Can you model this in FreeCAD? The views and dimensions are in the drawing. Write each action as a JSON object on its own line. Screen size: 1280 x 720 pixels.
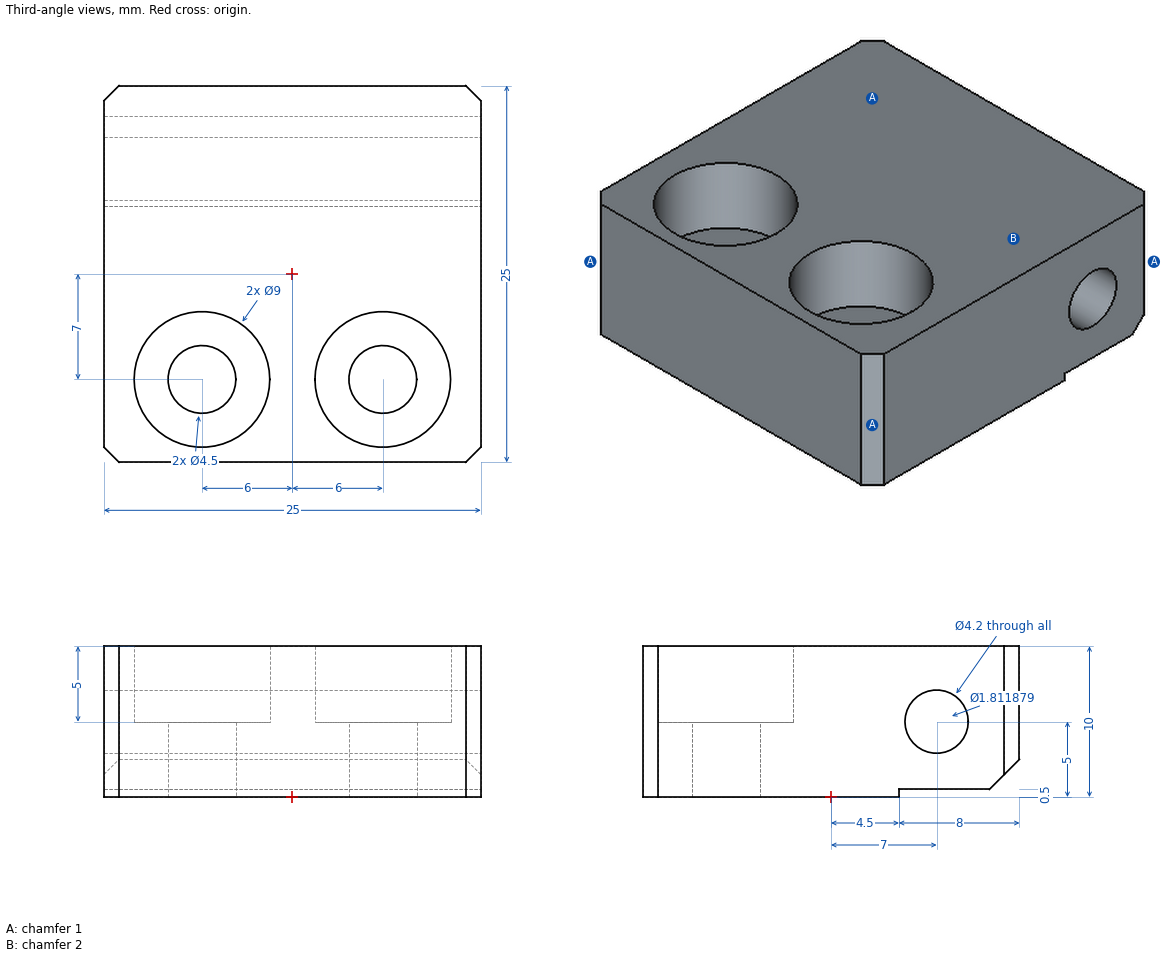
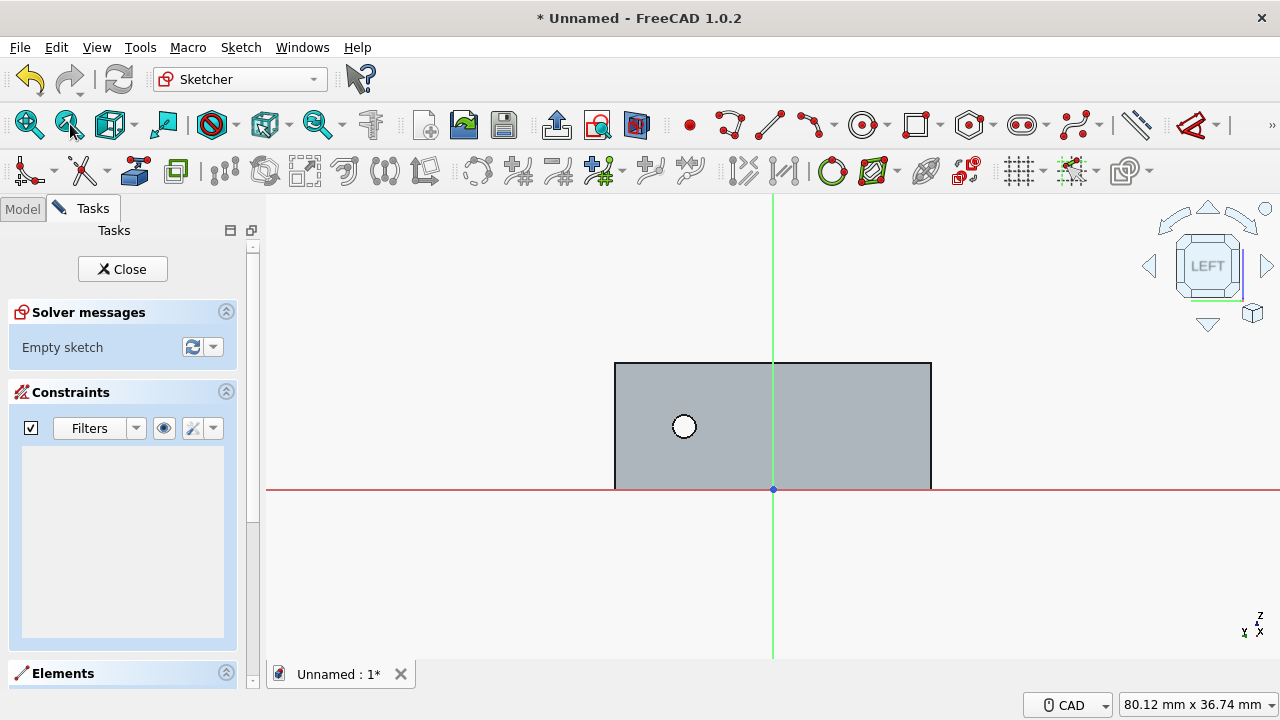
{"action": "scroll", "coordinate": [720, 453], "scroll_direction": "up", "scroll_amount": 6}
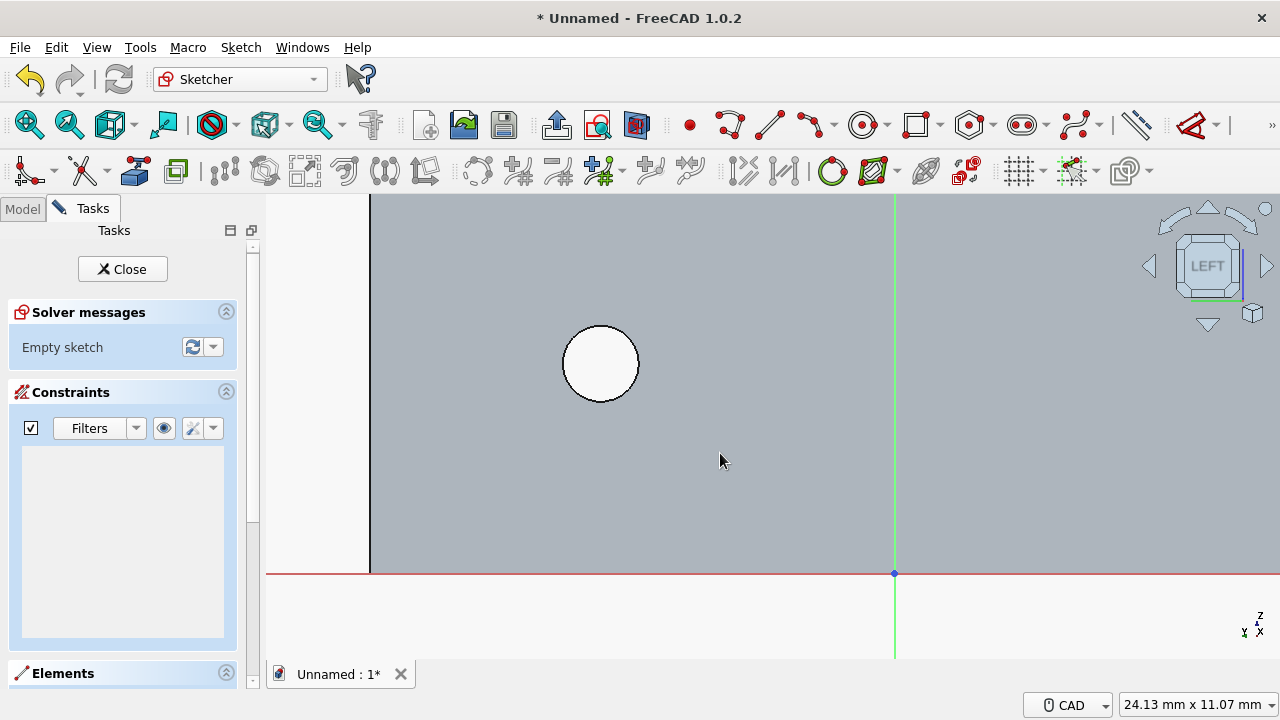
{"action": "key", "text": "g c"}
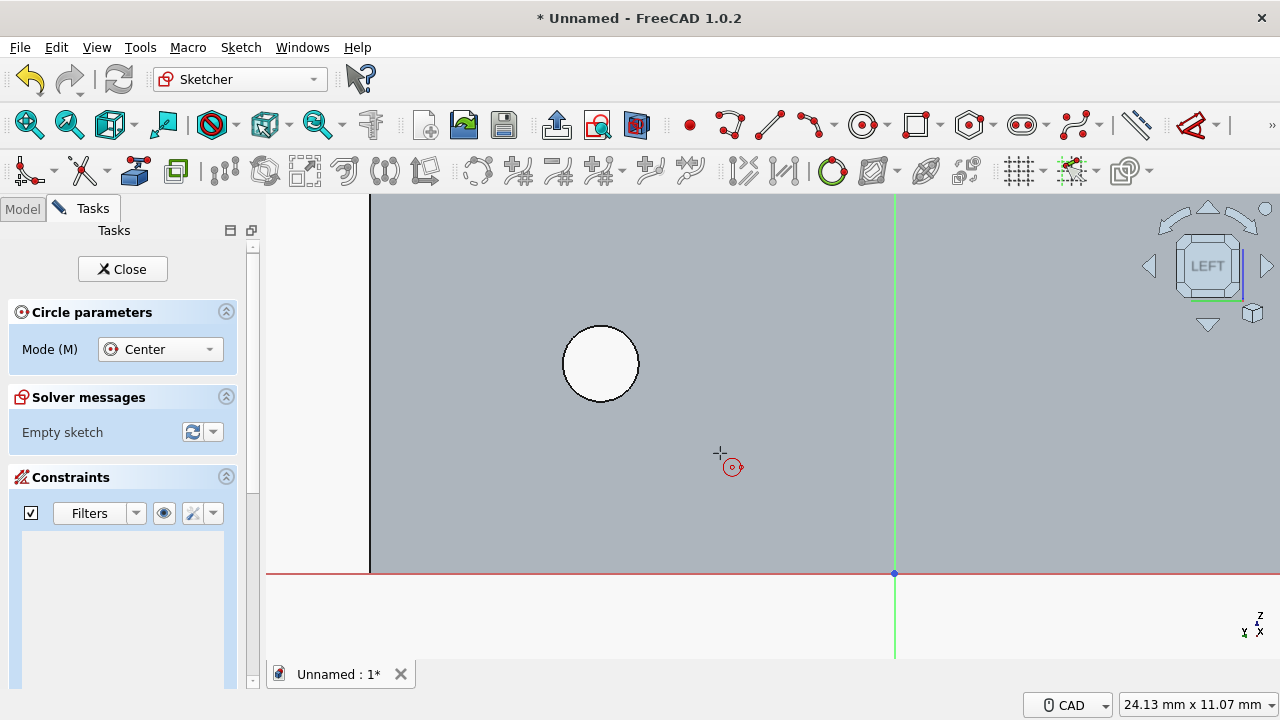
{"action": "left_click", "coordinate": [601, 364]}
{"action": "left_click", "coordinate": [663, 301]}
{"action": "key", "text": "Escape"}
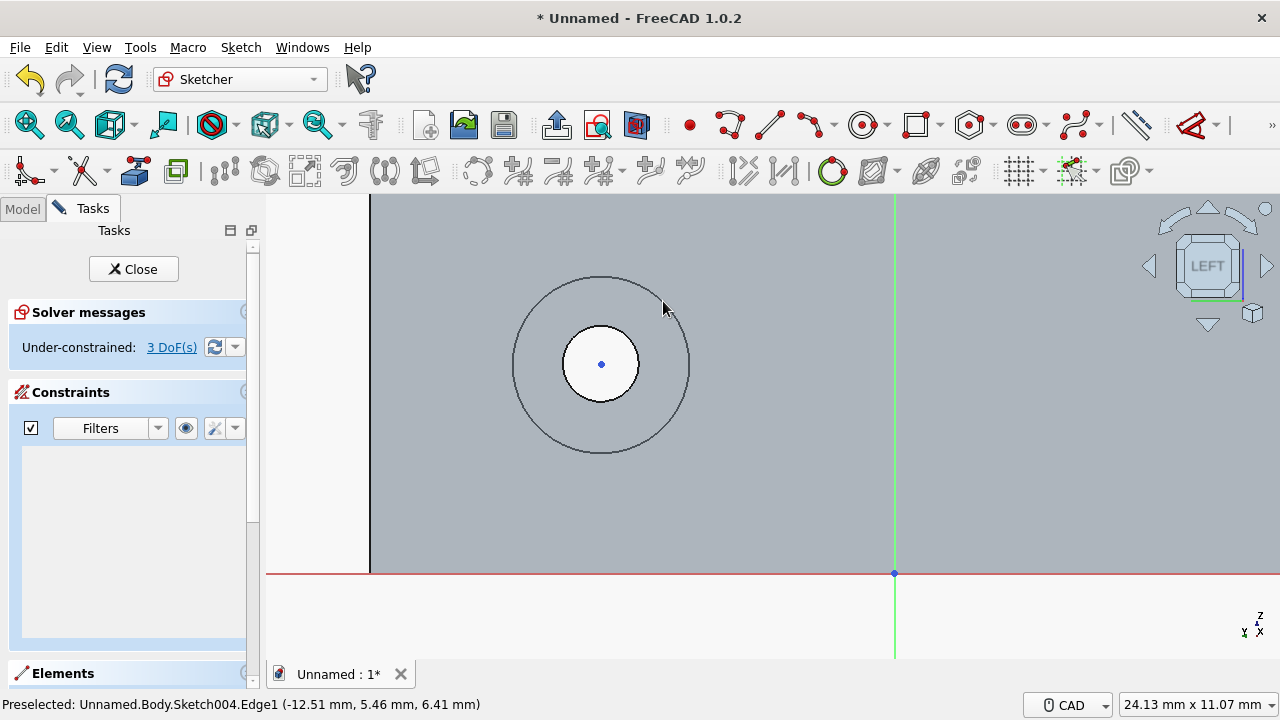
{"action": "key", "text": "d"}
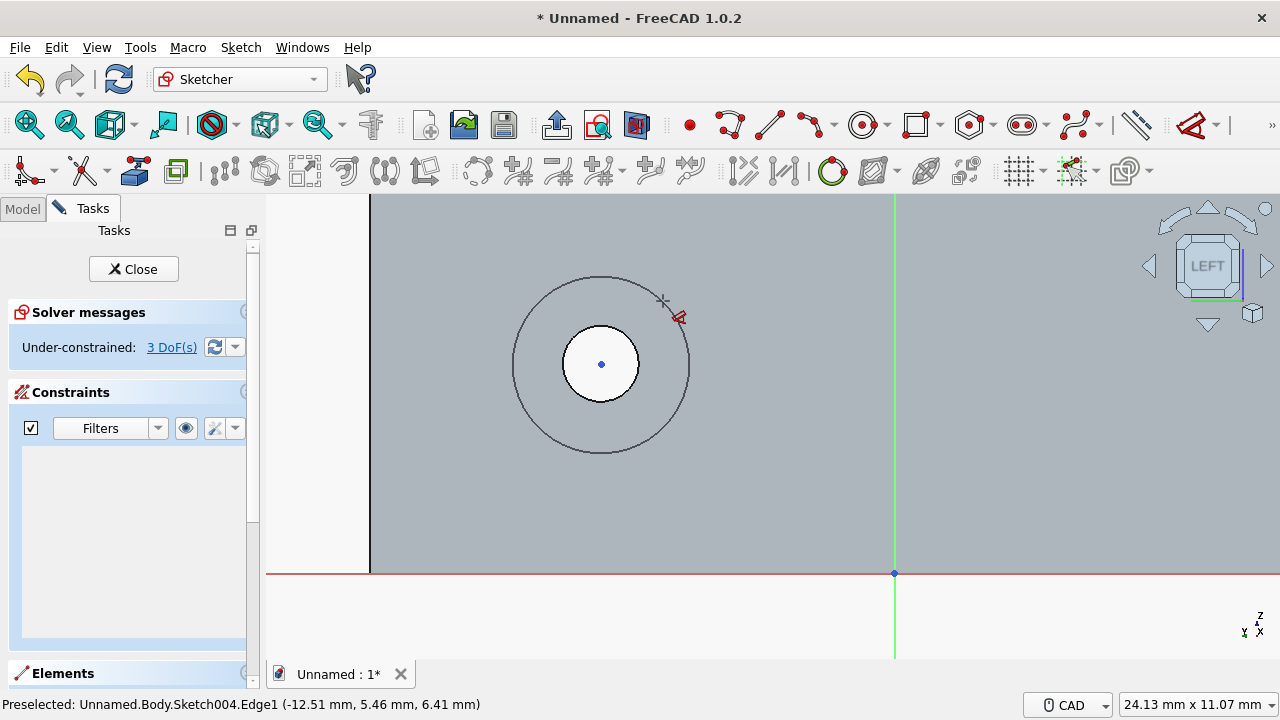
{"action": "left_click", "coordinate": [663, 302]}
{"action": "left_click", "coordinate": [685, 279]}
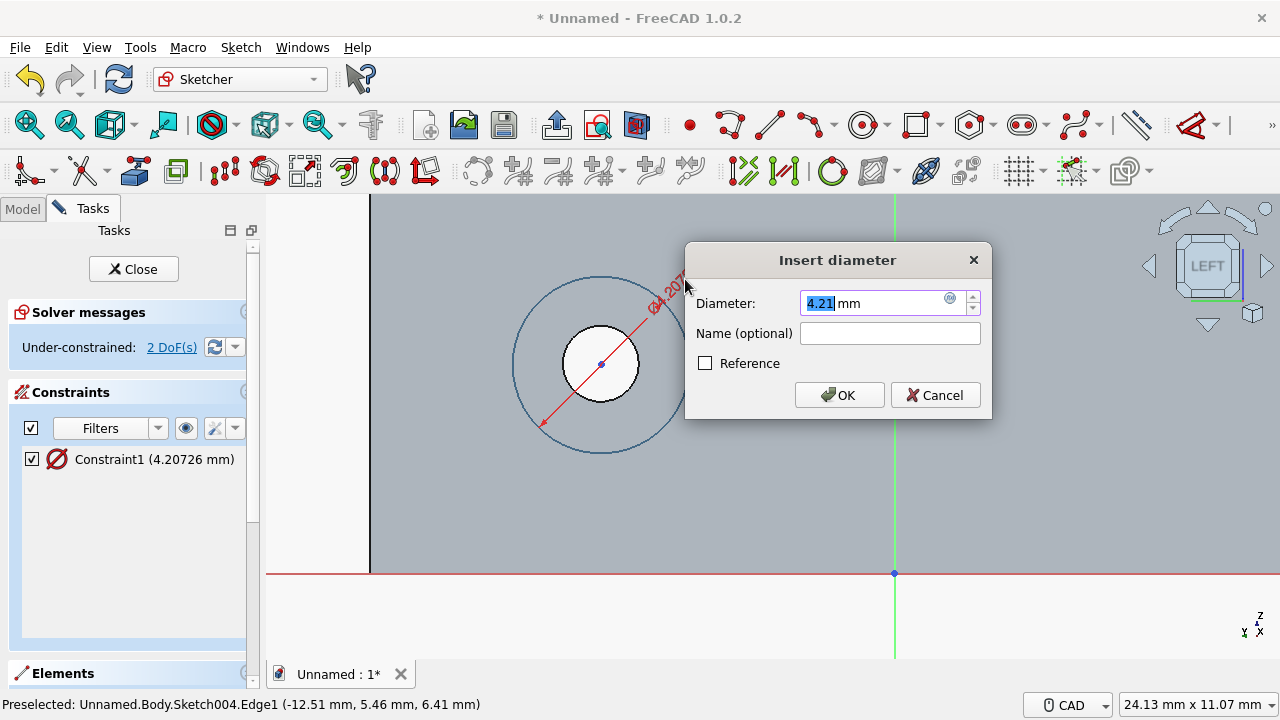
{"action": "type", "text": "4.2"}
{"action": "key", "text": "Return"}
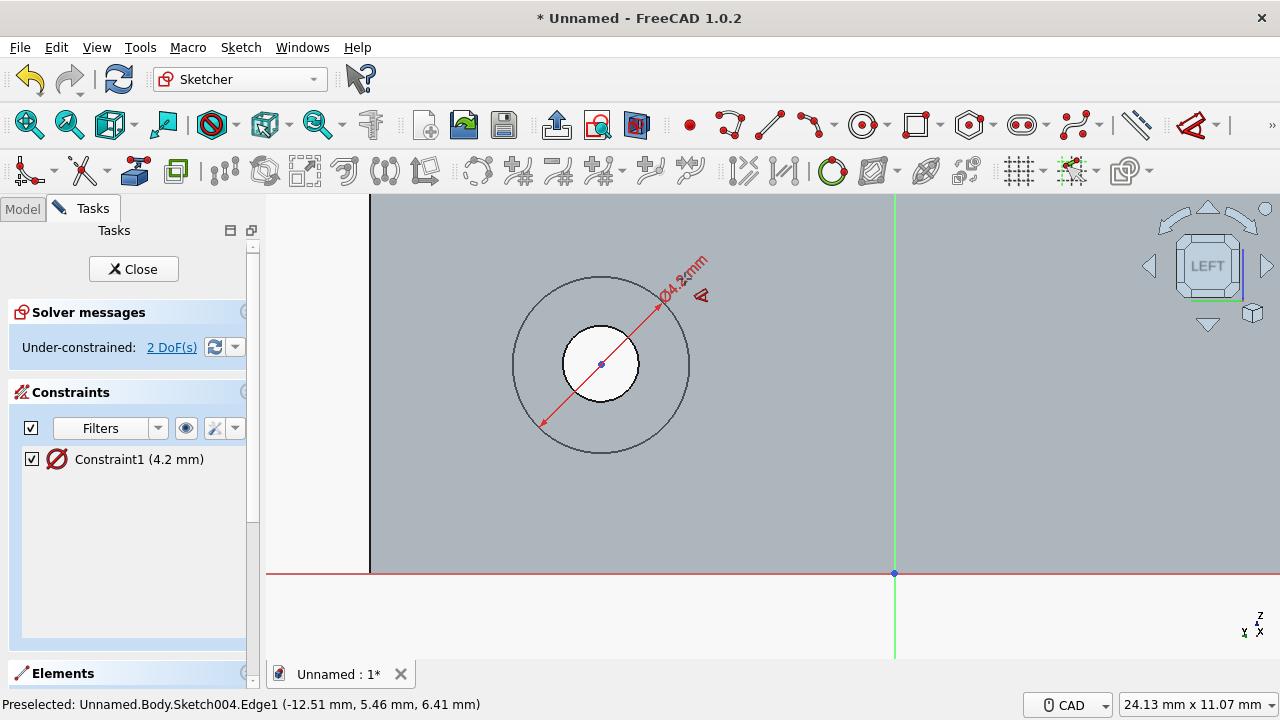
{"action": "left_click", "coordinate": [601, 365]}
{"action": "left_click", "coordinate": [748, 608]}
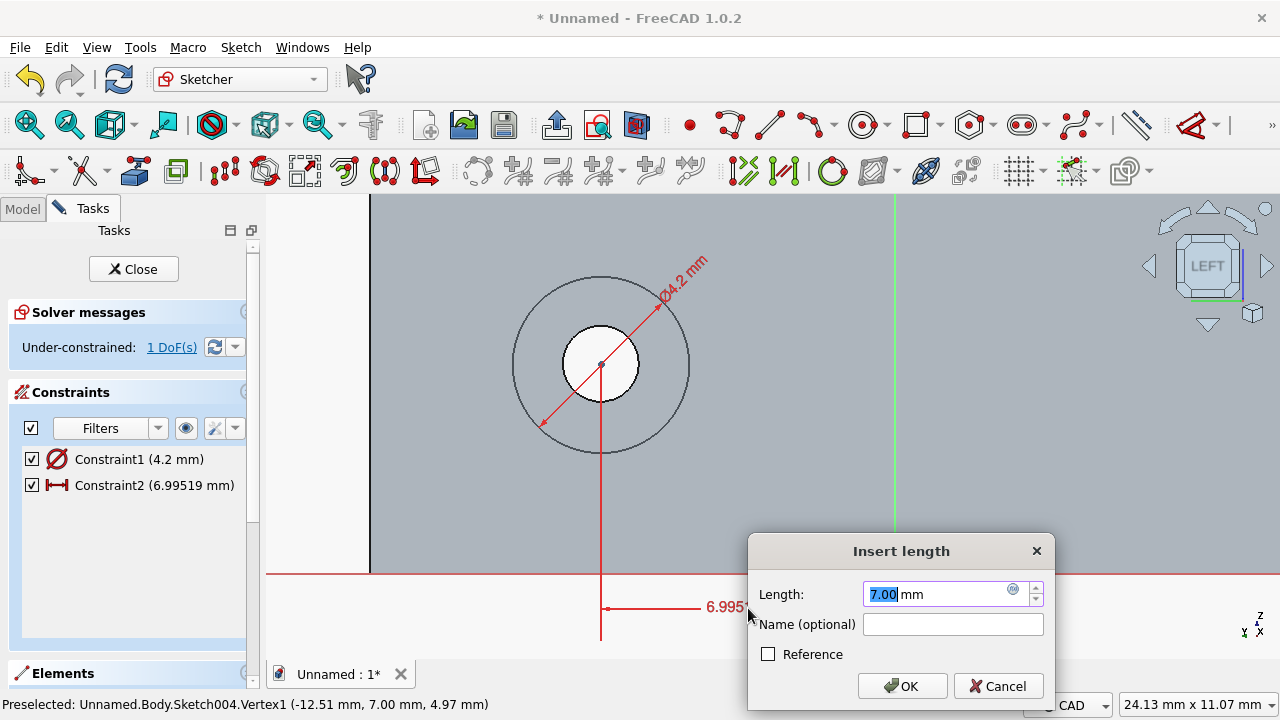
{"action": "type", "text": "7"}
{"action": "key", "text": "Return"}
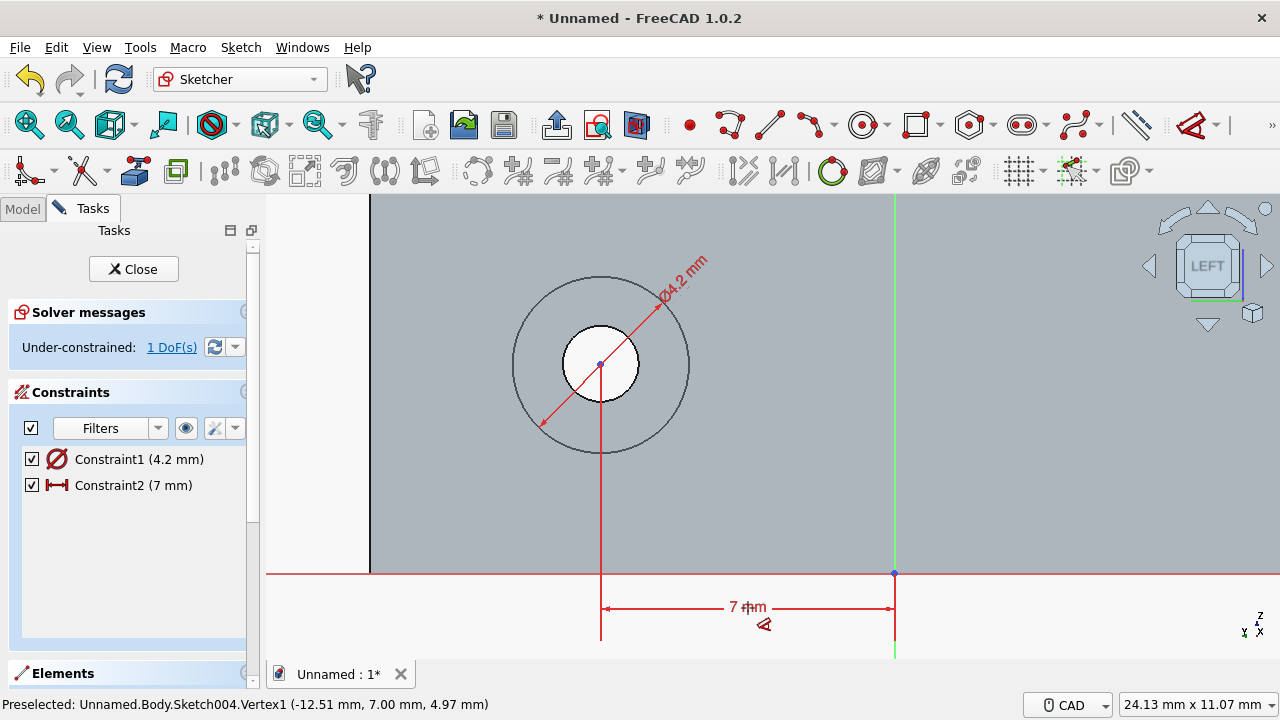
{"action": "left_click", "coordinate": [601, 365]}
{"action": "left_click", "coordinate": [929, 469]}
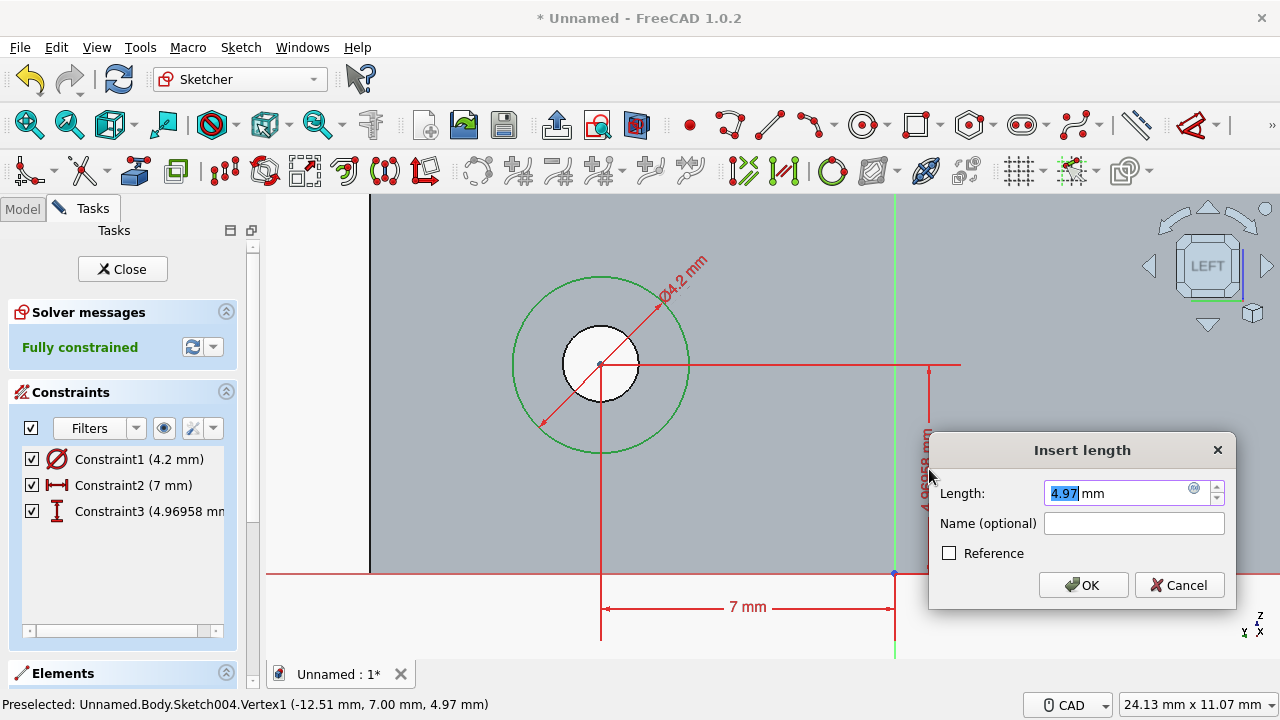
{"action": "type", "text": "5"}
{"action": "key", "text": "Return"}
{"action": "key", "text": "Escape"}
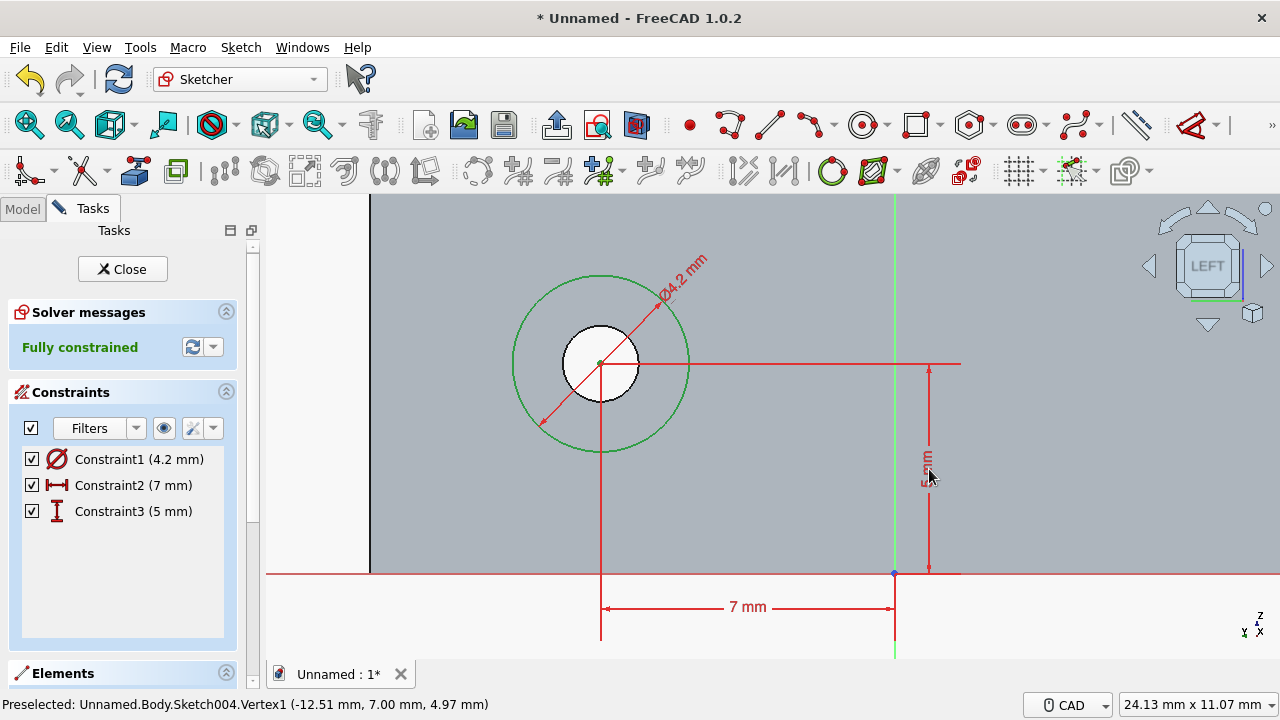
{"action": "left_click", "coordinate": [123, 269]}